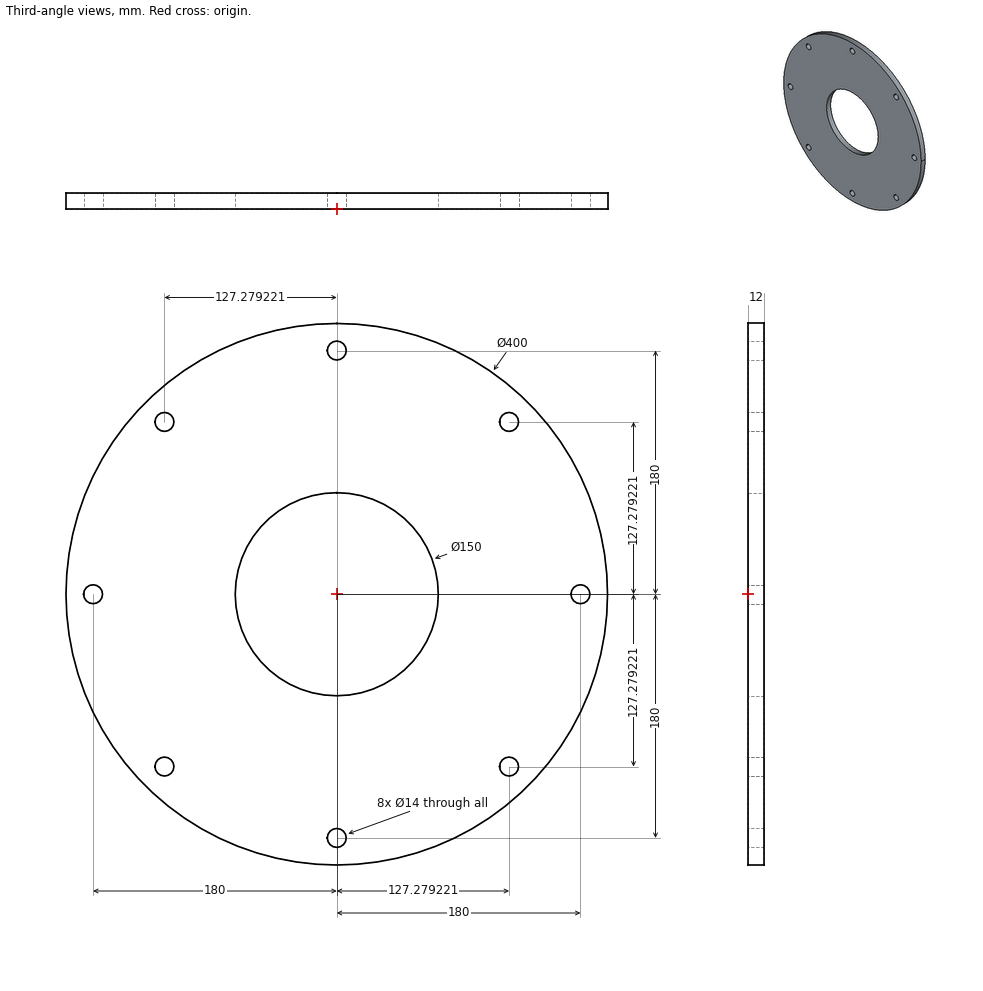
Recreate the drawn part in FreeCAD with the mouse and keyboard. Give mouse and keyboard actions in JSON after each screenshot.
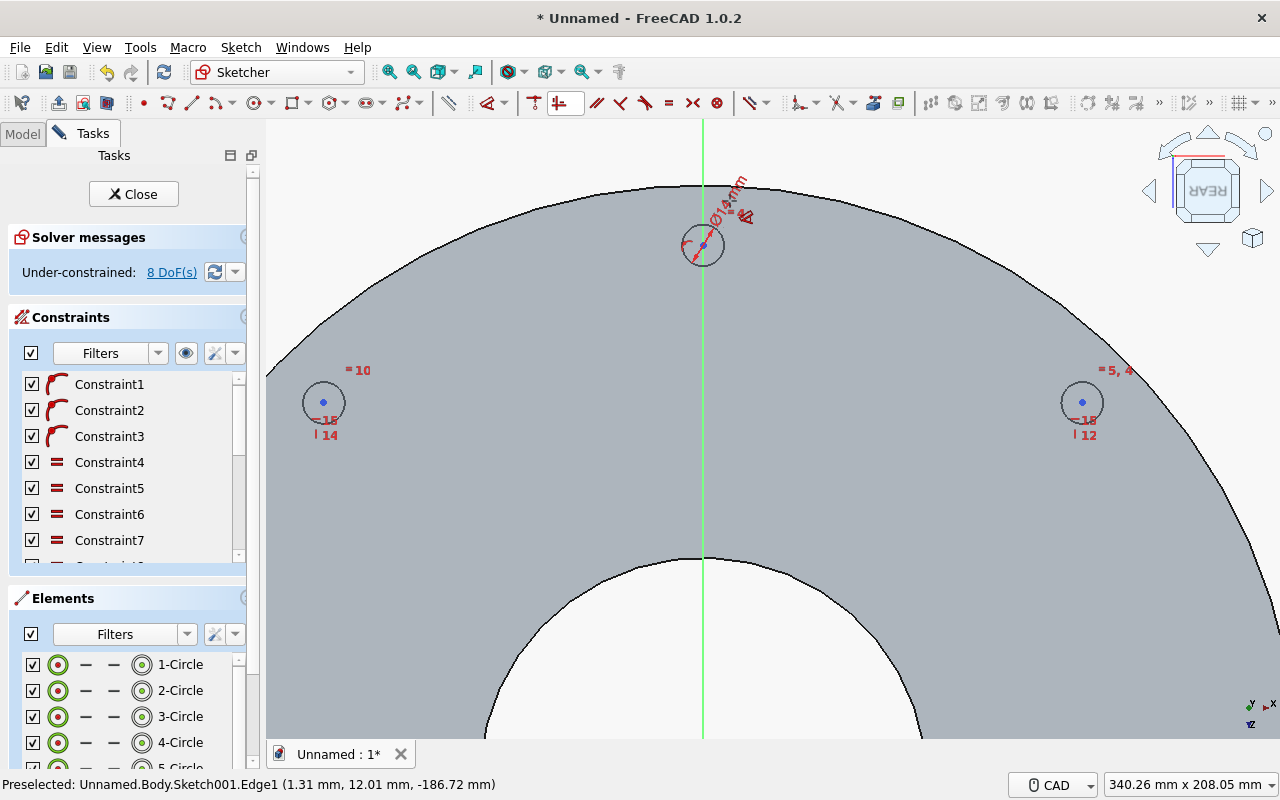
{"action": "left_click", "coordinate": [703, 245]}
{"action": "left_click", "coordinate": [737, 478]}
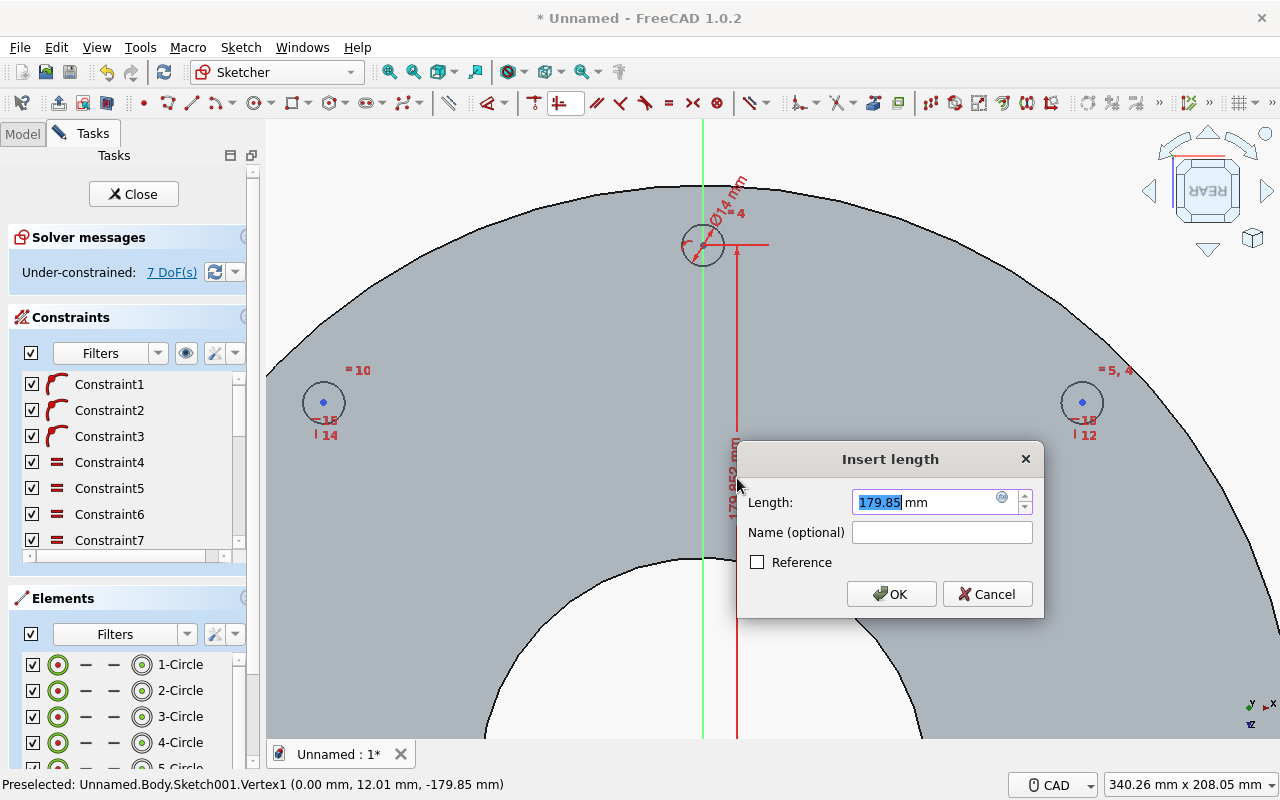
{"action": "type", "text": "180"}
{"action": "key", "text": "Return"}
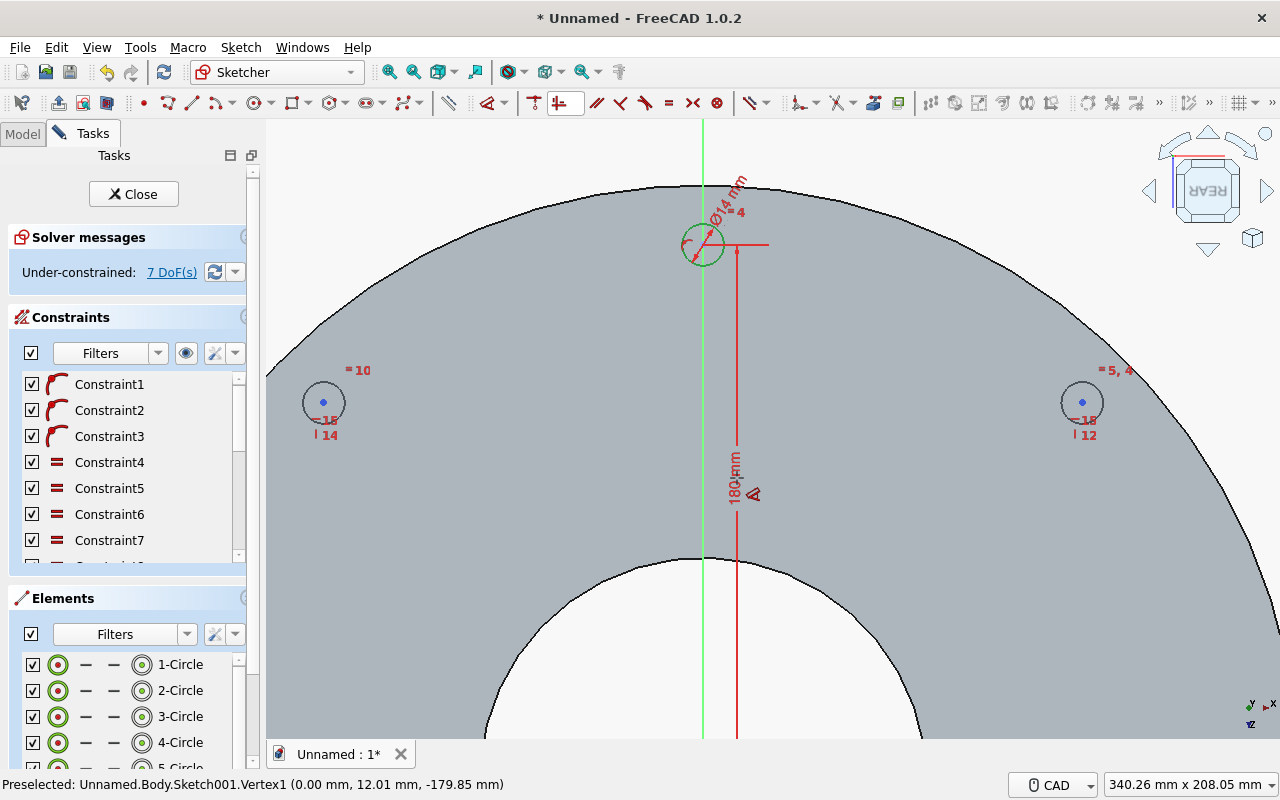
{"action": "scroll", "coordinate": [705, 224], "scroll_direction": "down", "scroll_amount": 5}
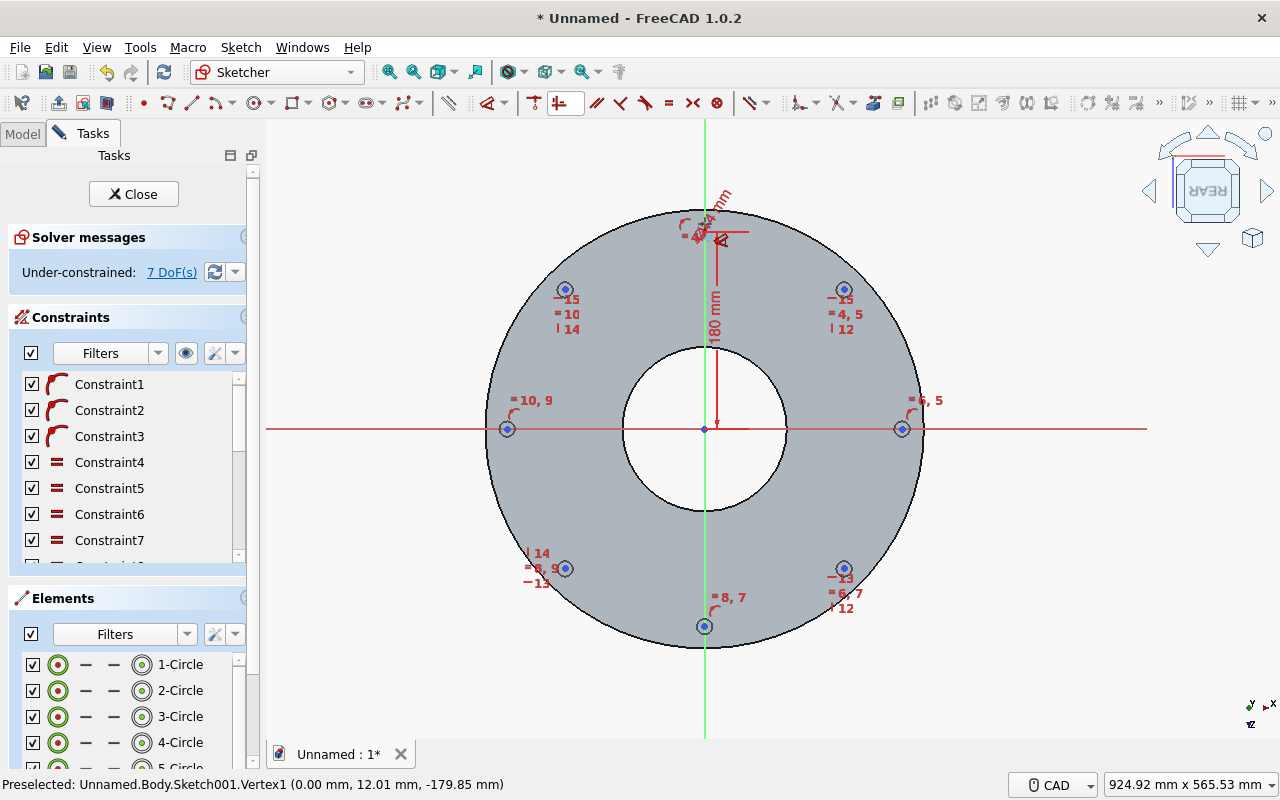
{"action": "left_click", "coordinate": [902, 429]}
{"action": "left_click", "coordinate": [803, 463]}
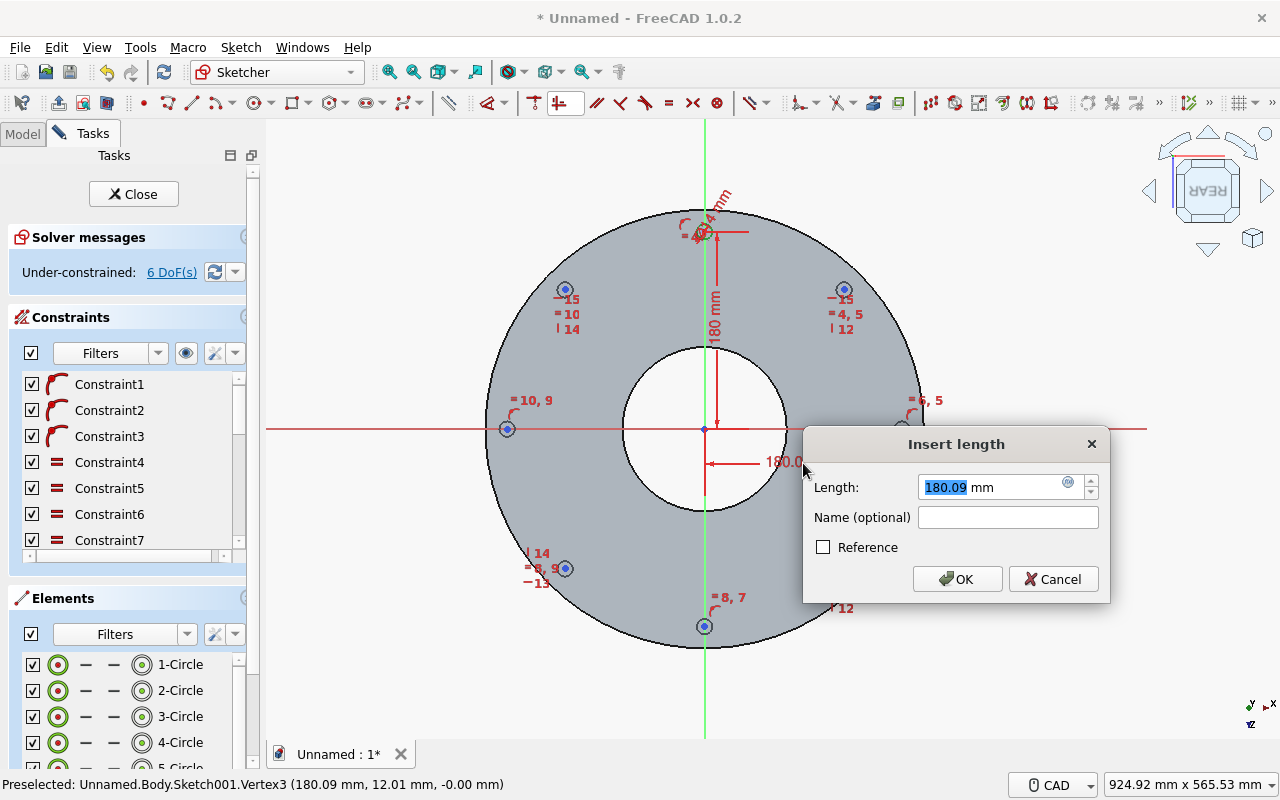
{"action": "type", "text": "180"}
{"action": "key", "text": "Return"}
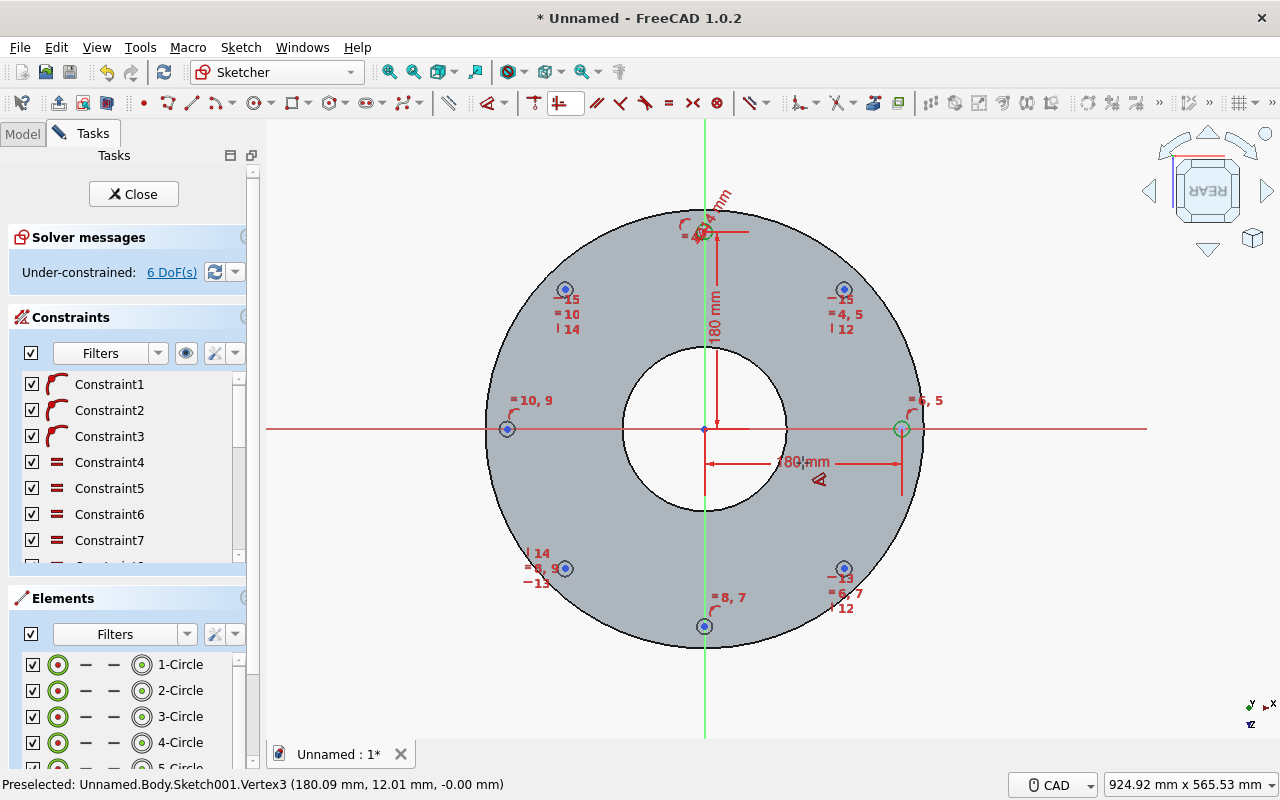
{"action": "left_click", "coordinate": [705, 627]}
{"action": "left_click", "coordinate": [739, 528]}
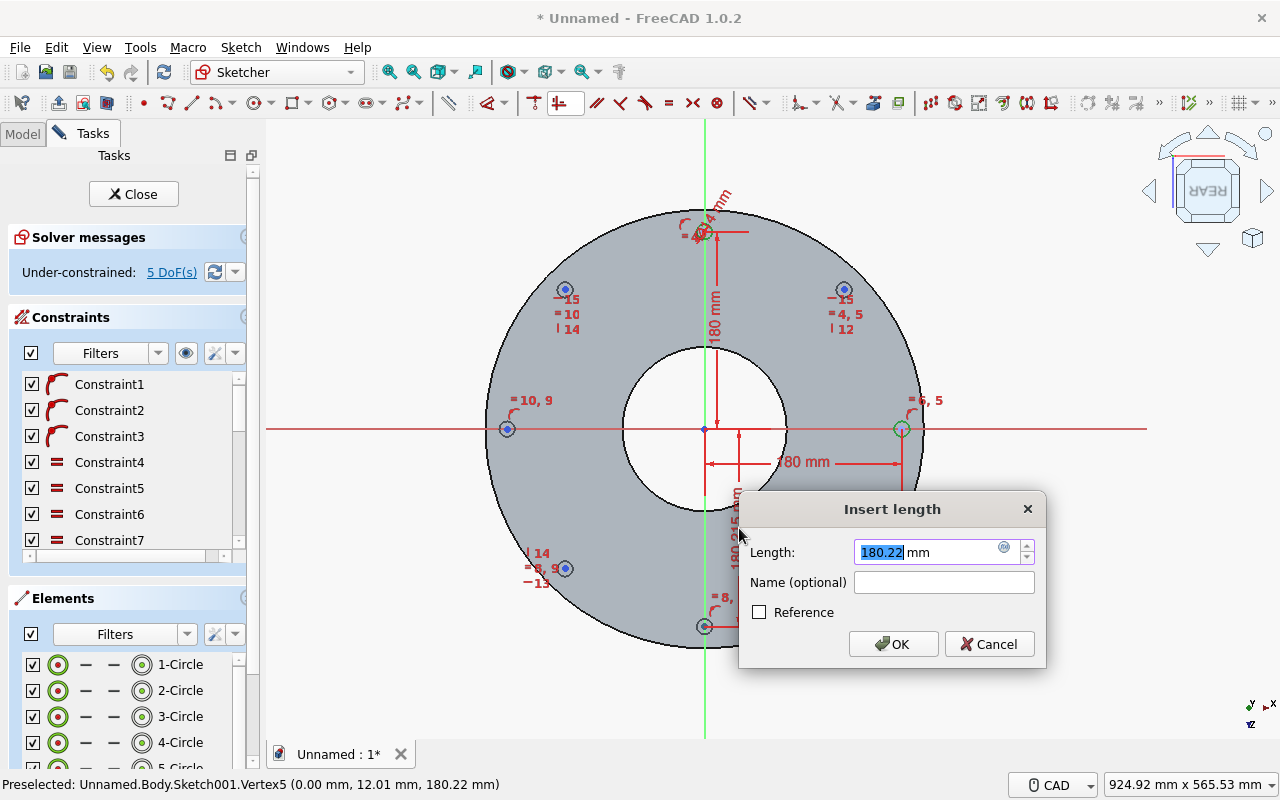
{"action": "type", "text": "180"}
{"action": "key", "text": "Return"}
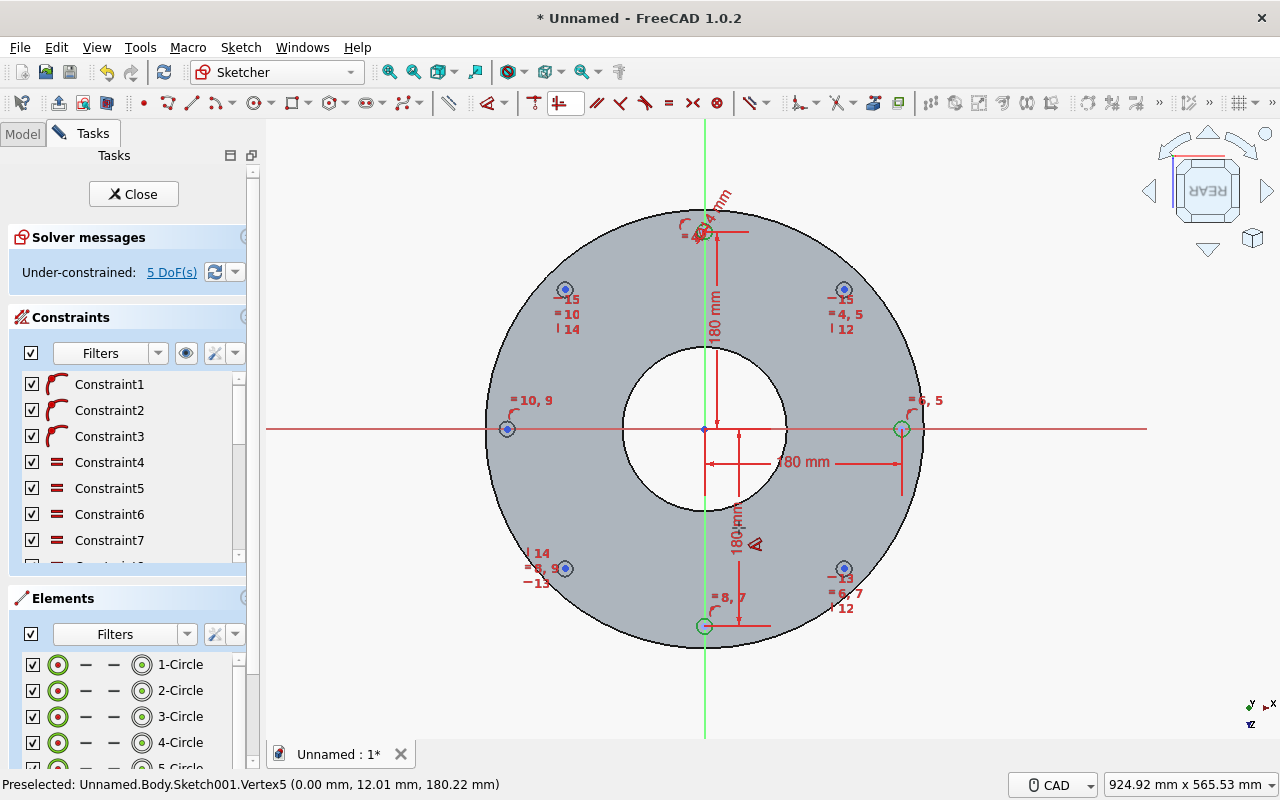
{"action": "left_click", "coordinate": [507, 429]}
{"action": "left_click", "coordinate": [606, 463]}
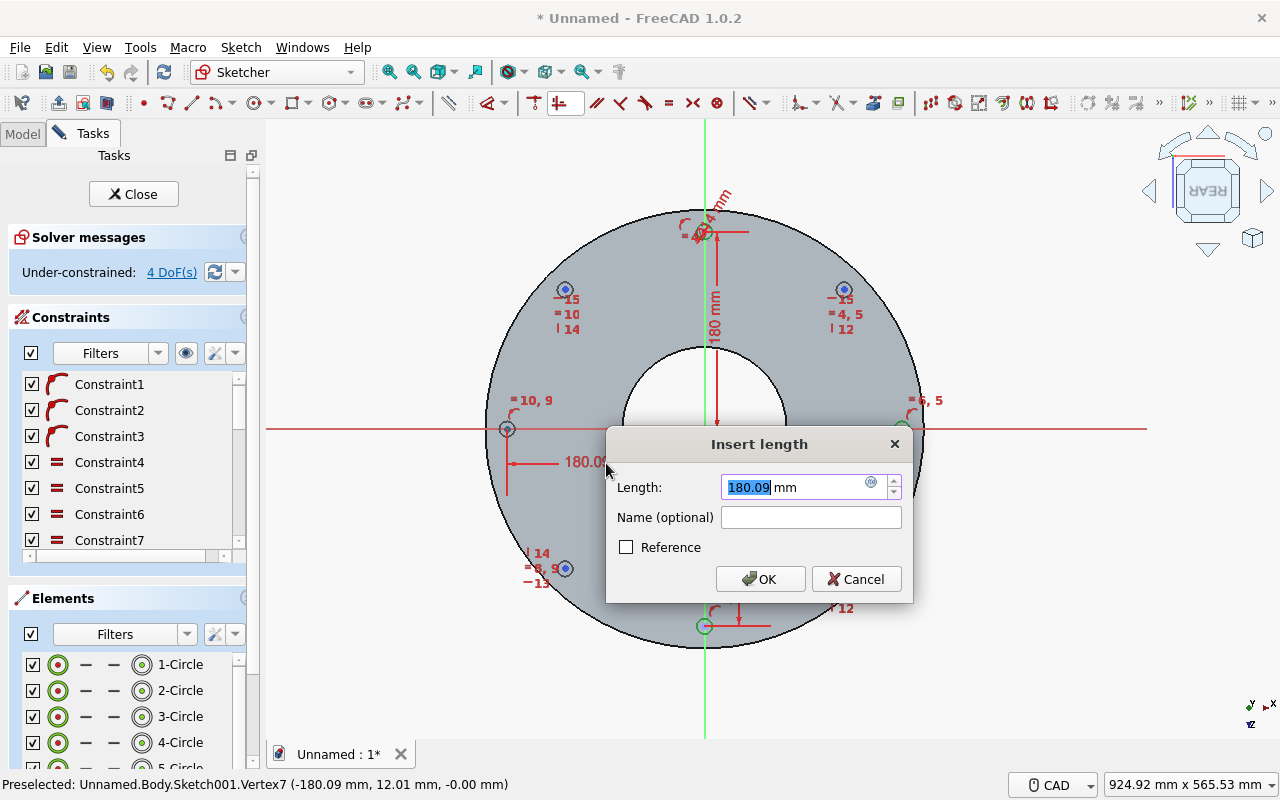
{"action": "type", "text": "180"}
{"action": "key", "text": "Return"}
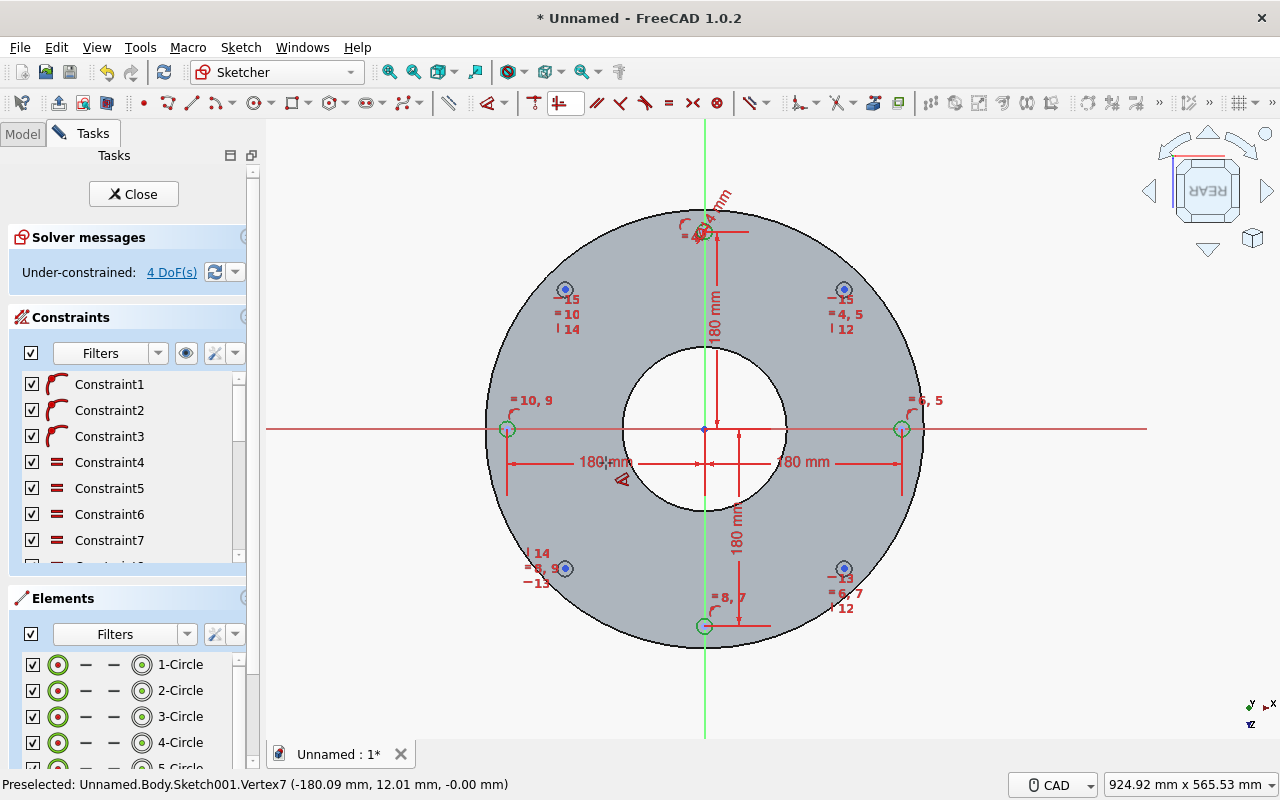
{"action": "left_click", "coordinate": [844, 290]}
{"action": "left_click", "coordinate": [774, 256]}